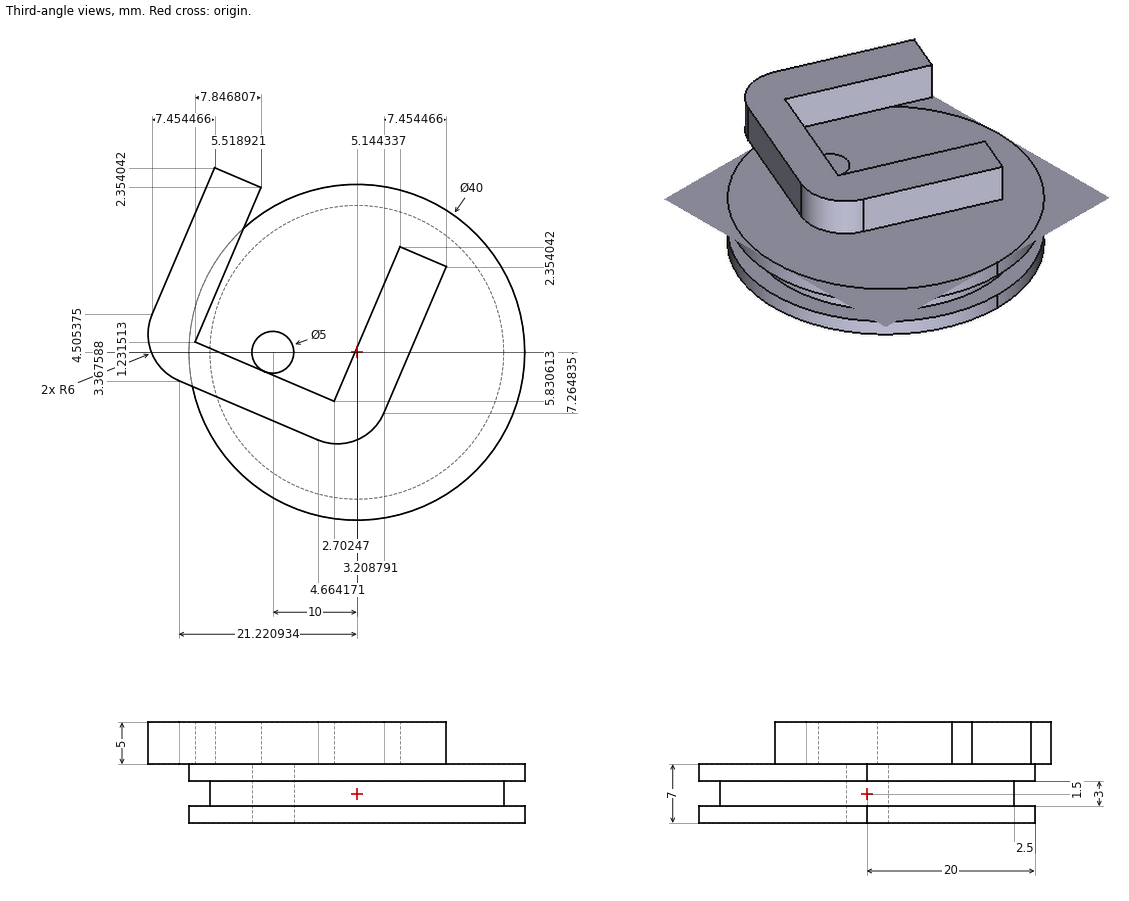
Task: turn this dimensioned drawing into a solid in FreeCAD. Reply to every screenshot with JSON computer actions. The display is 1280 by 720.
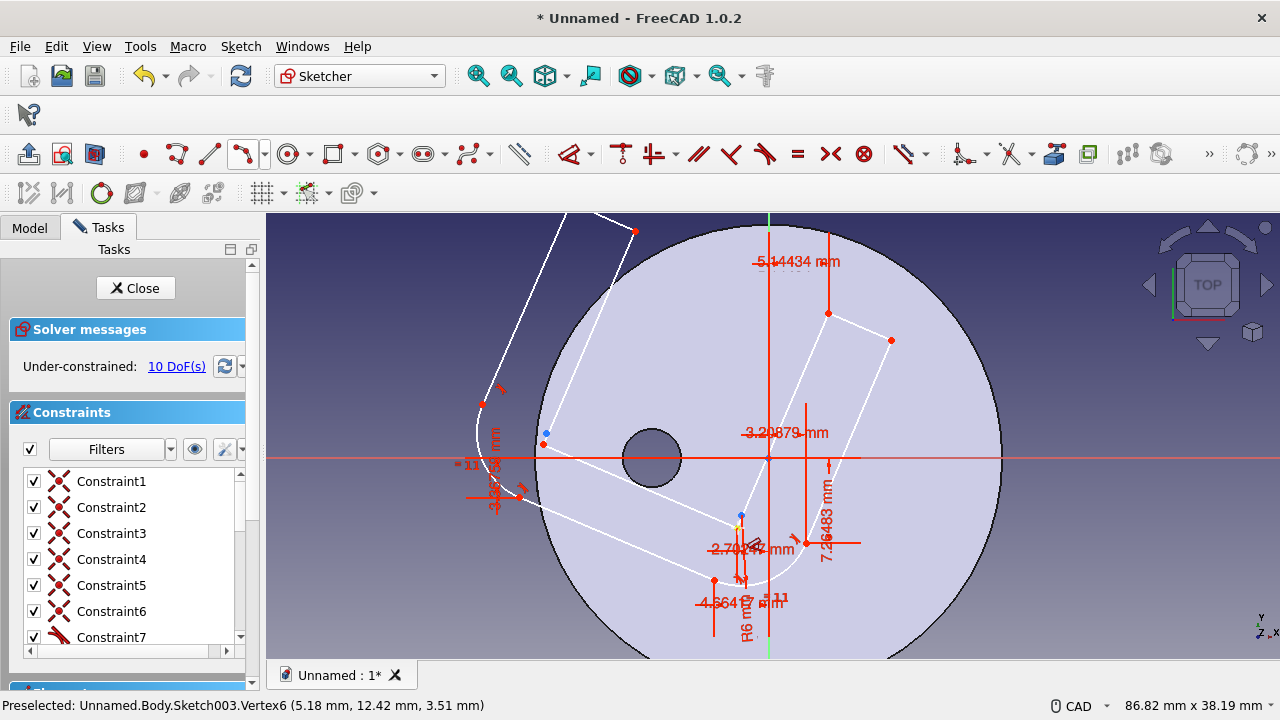
{"action": "left_click", "coordinate": [737, 528]}
{"action": "left_click", "coordinate": [803, 493]}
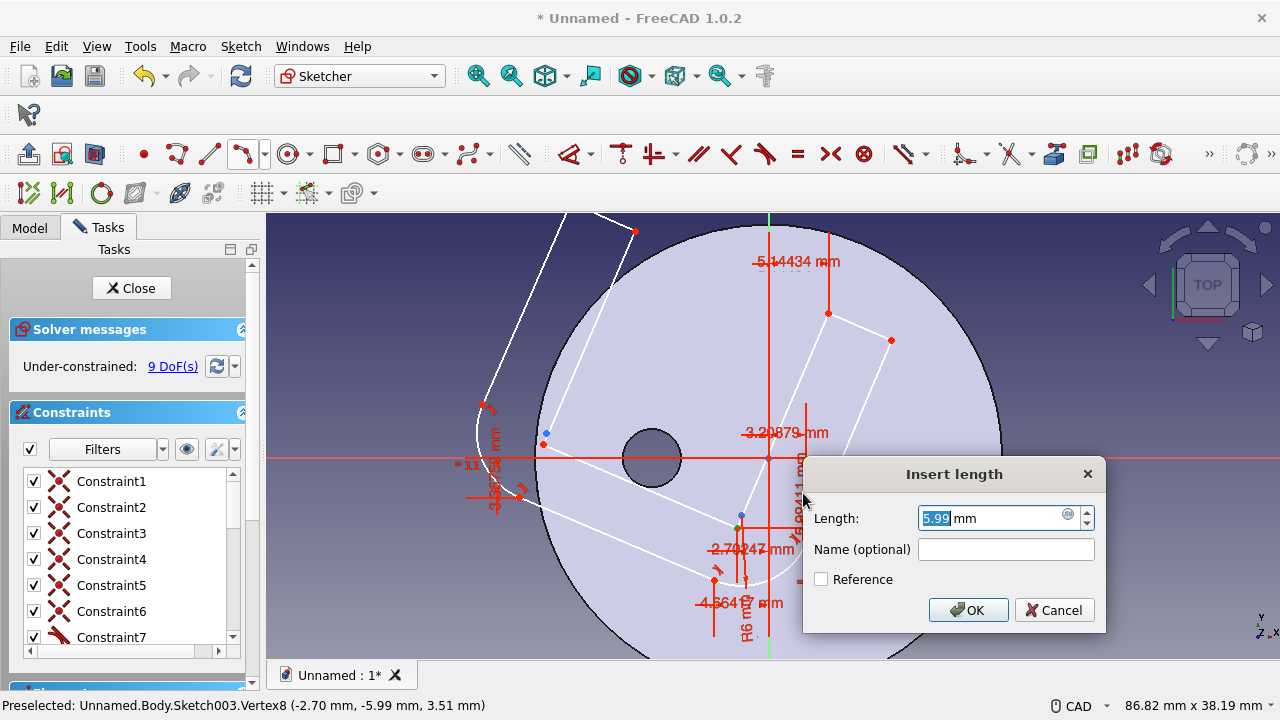
{"action": "type", "text": "5.830613"}
{"action": "key", "text": "Return"}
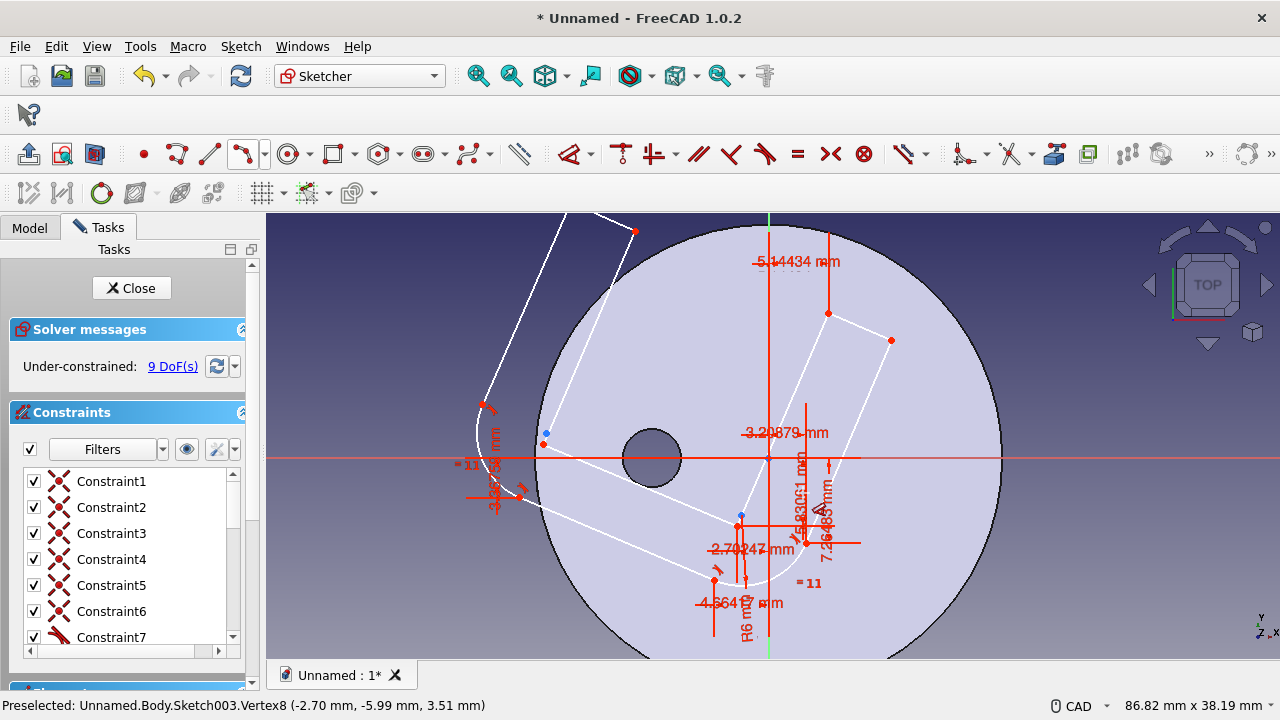
{"action": "scroll", "coordinate": [543, 445], "scroll_direction": "up", "scroll_amount": 6}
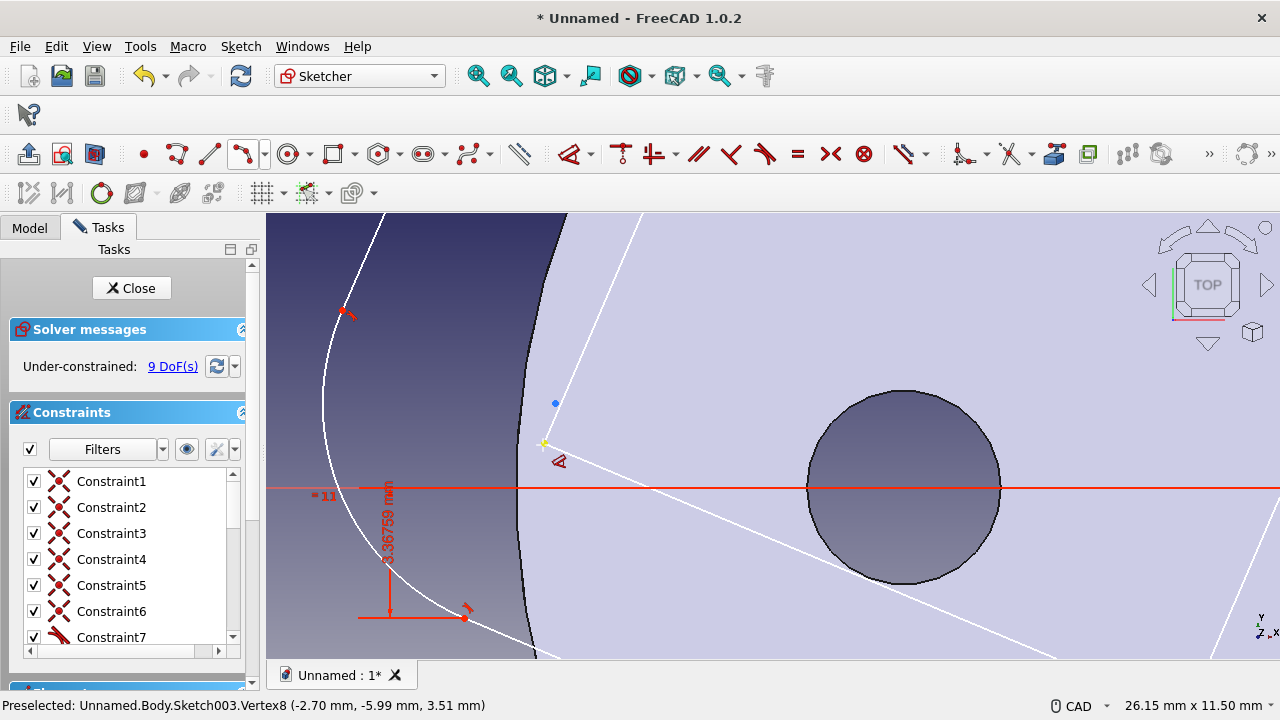
{"action": "left_click", "coordinate": [544, 444]}
{"action": "left_click", "coordinate": [510, 466]}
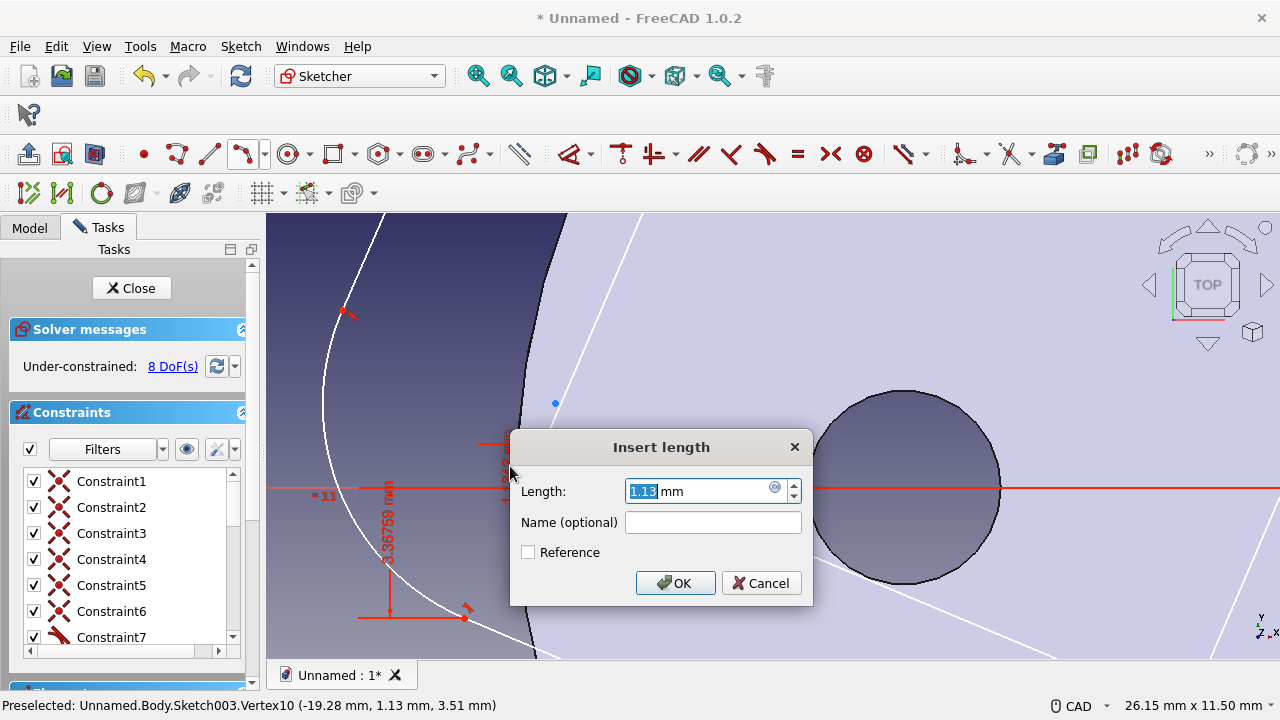
{"action": "type", "text": "1.231513"}
{"action": "key", "text": "Return"}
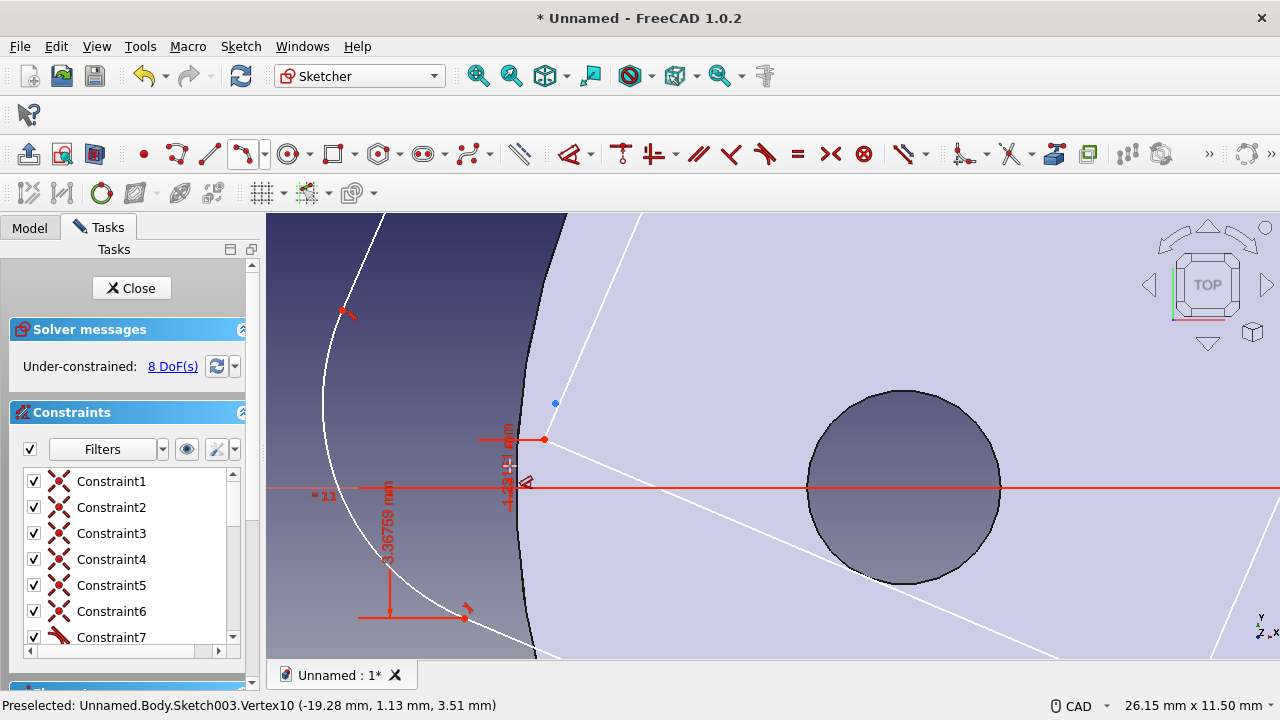
{"action": "scroll", "coordinate": [624, 479], "scroll_direction": "down", "scroll_amount": 8}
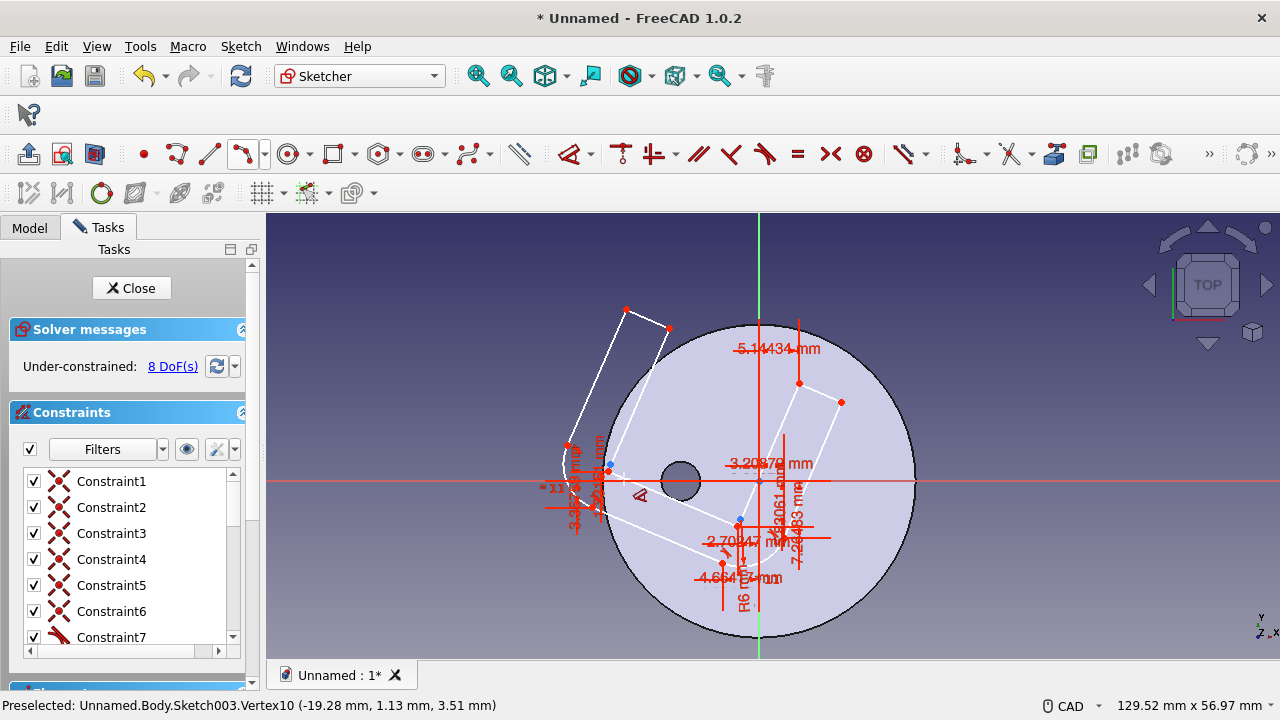
{"action": "left_click", "coordinate": [567, 446]}
{"action": "left_click", "coordinate": [533, 455]}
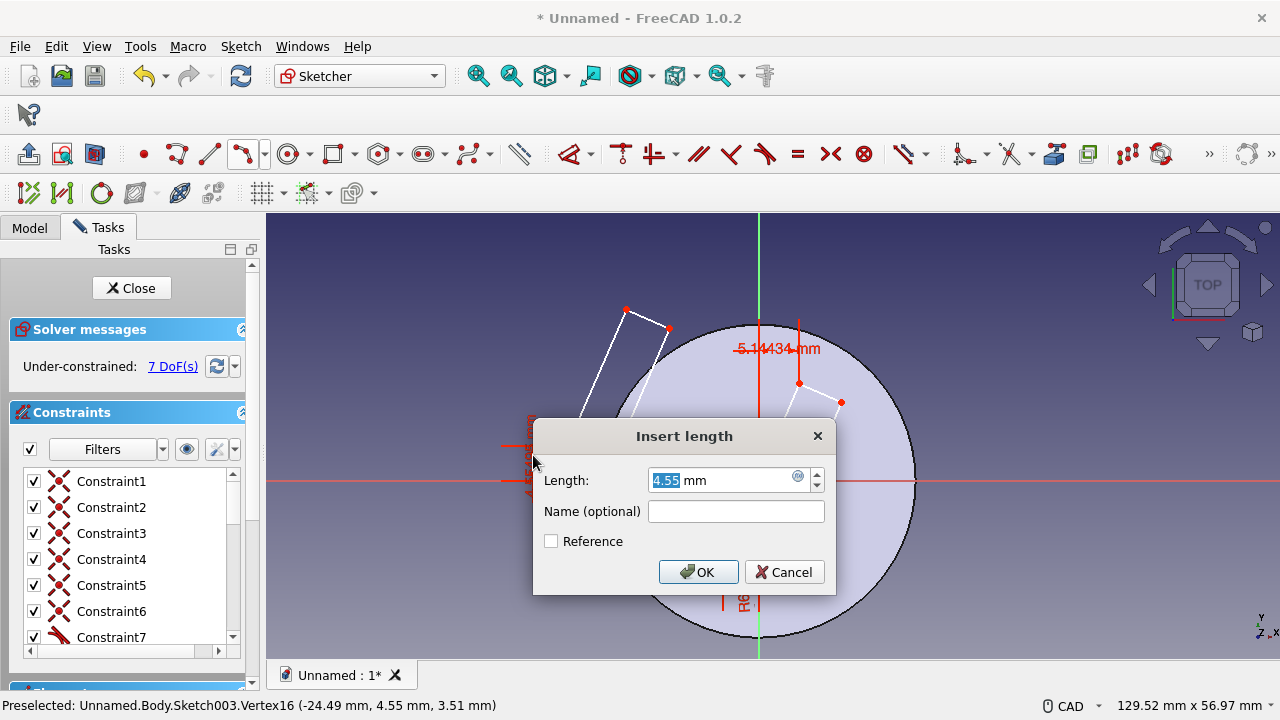
{"action": "type", "text": "4.505375"}
{"action": "key", "text": "Return"}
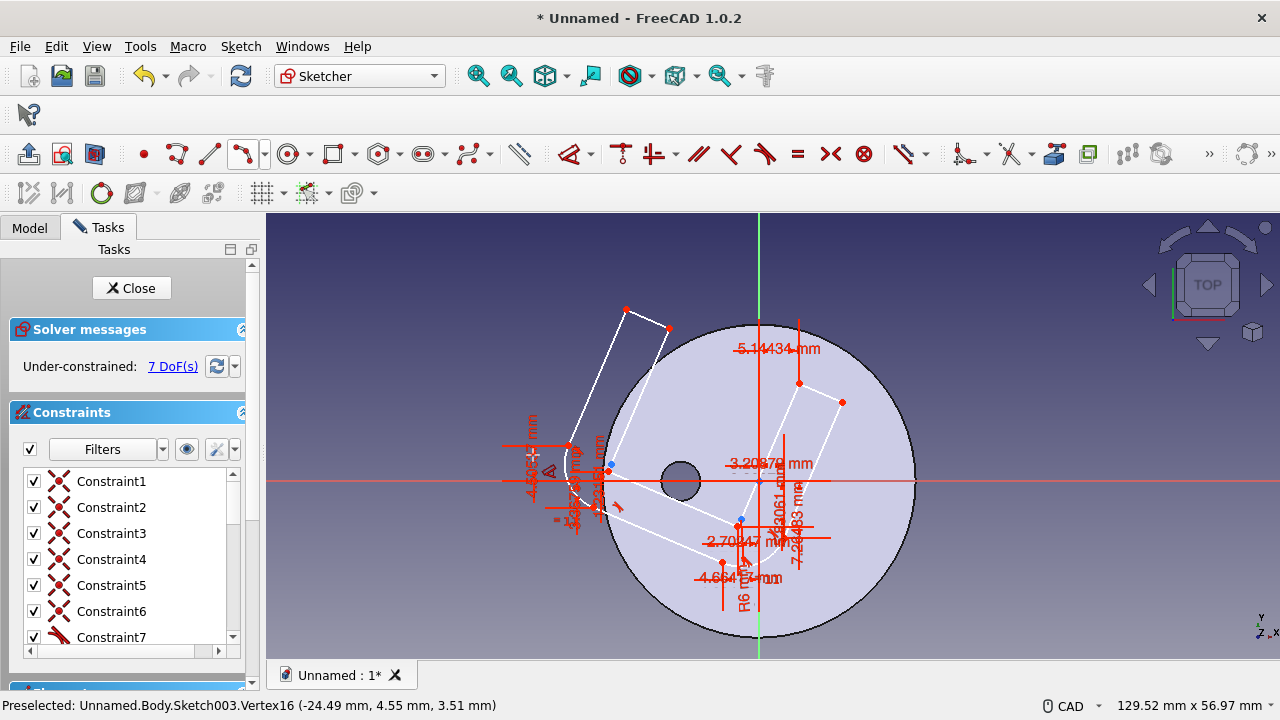
{"action": "left_click", "coordinate": [802, 497]}
{"action": "left_click", "coordinate": [827, 572]}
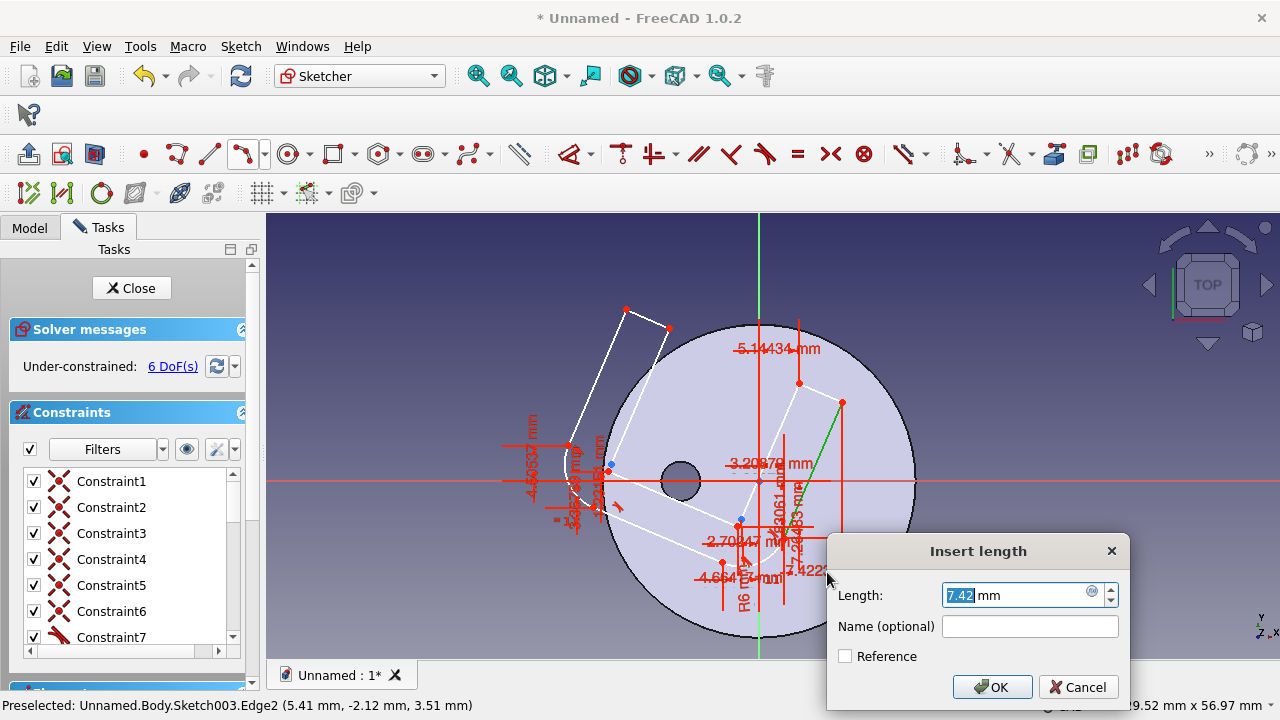
{"action": "type", "text": "7.454466"}
{"action": "key", "text": "Return"}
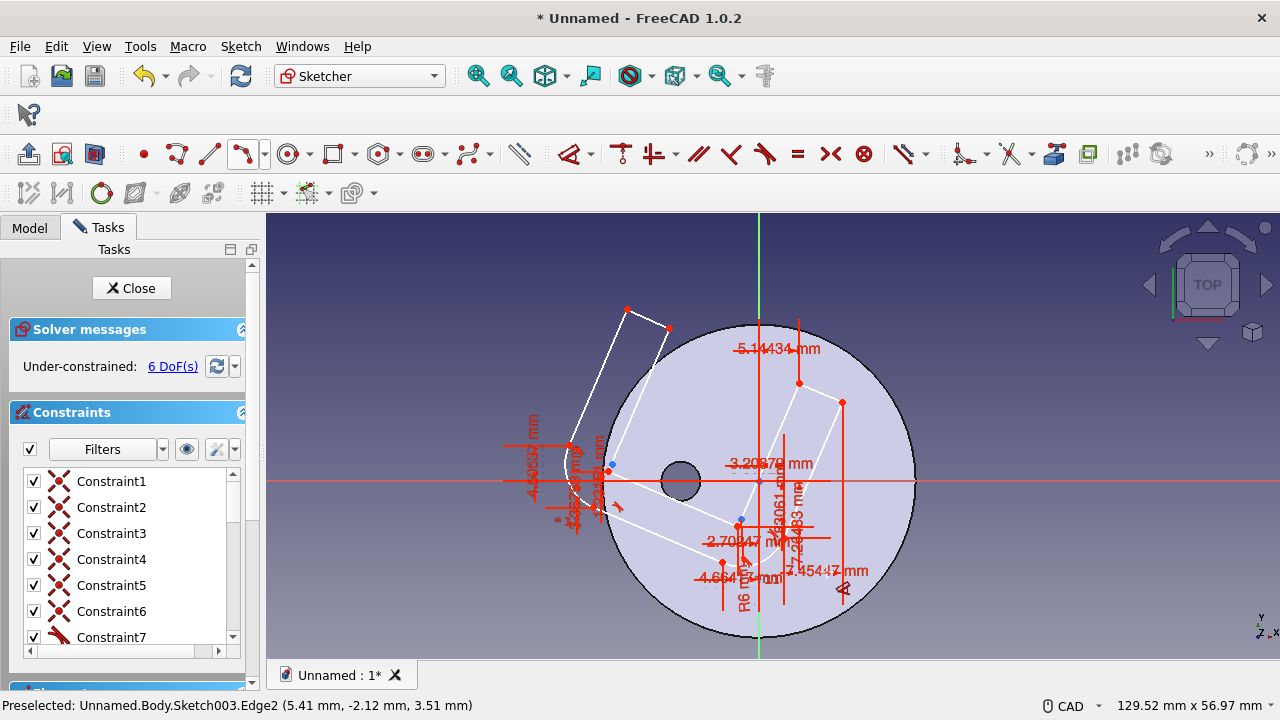
{"action": "scroll", "coordinate": [830, 397], "scroll_direction": "up", "scroll_amount": 4}